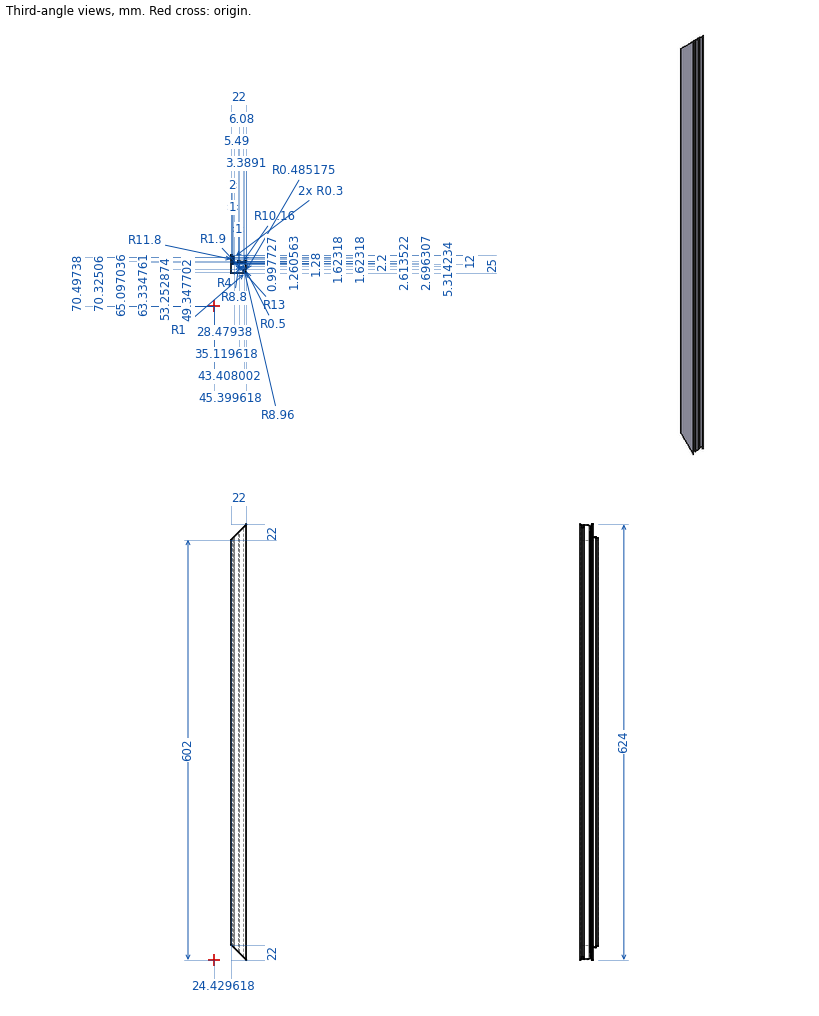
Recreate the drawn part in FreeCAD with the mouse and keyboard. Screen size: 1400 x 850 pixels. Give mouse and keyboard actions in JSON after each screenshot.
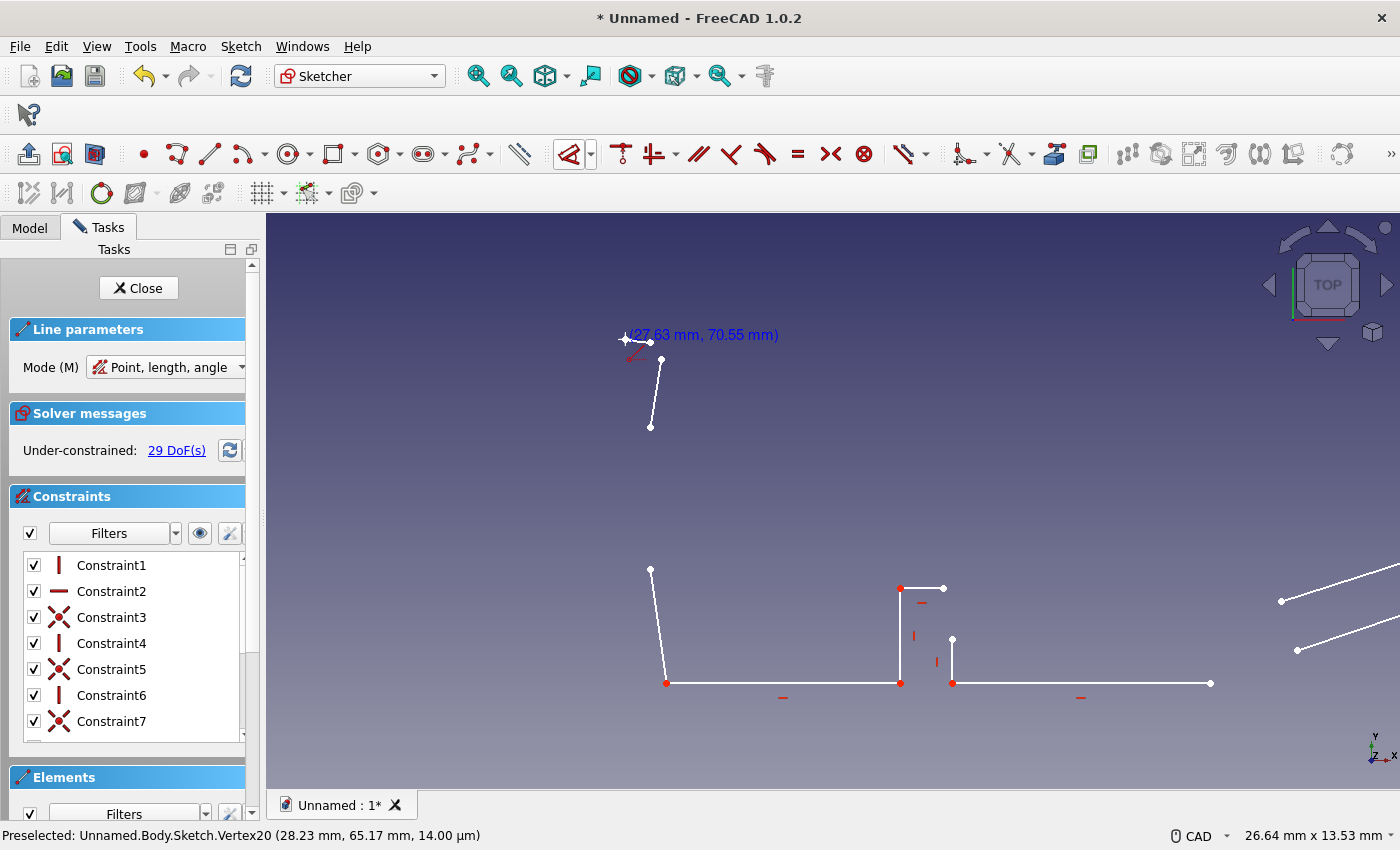
{"action": "left_click", "coordinate": [611, 350]}
{"action": "left_click", "coordinate": [601, 419]}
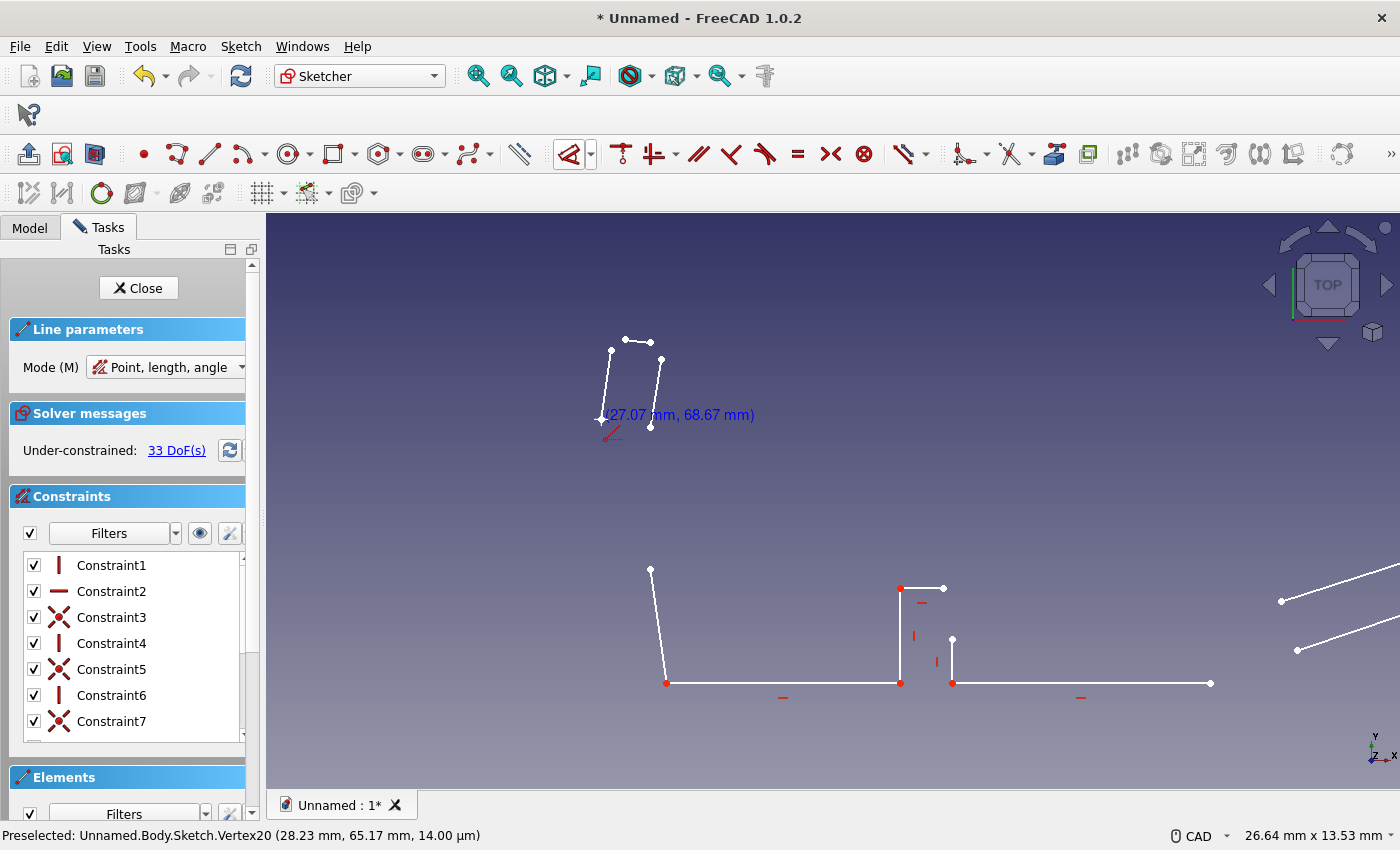
{"action": "key", "text": "g m"}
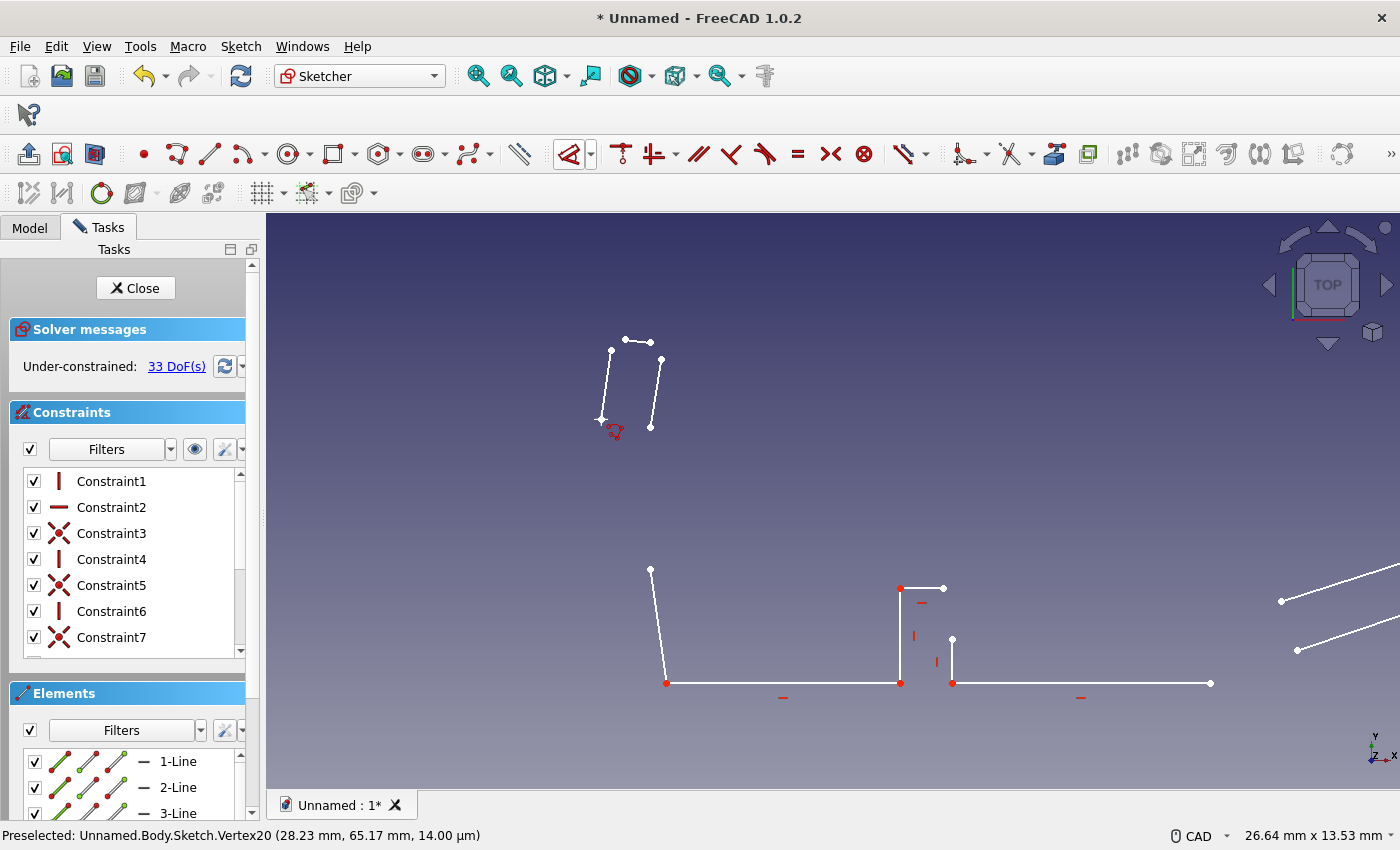
{"action": "left_click", "coordinate": [601, 572]}
{"action": "left_click", "coordinate": [616, 684]}
{"action": "left_click", "coordinate": [616, 738]}
{"action": "left_click", "coordinate": [574, 738]}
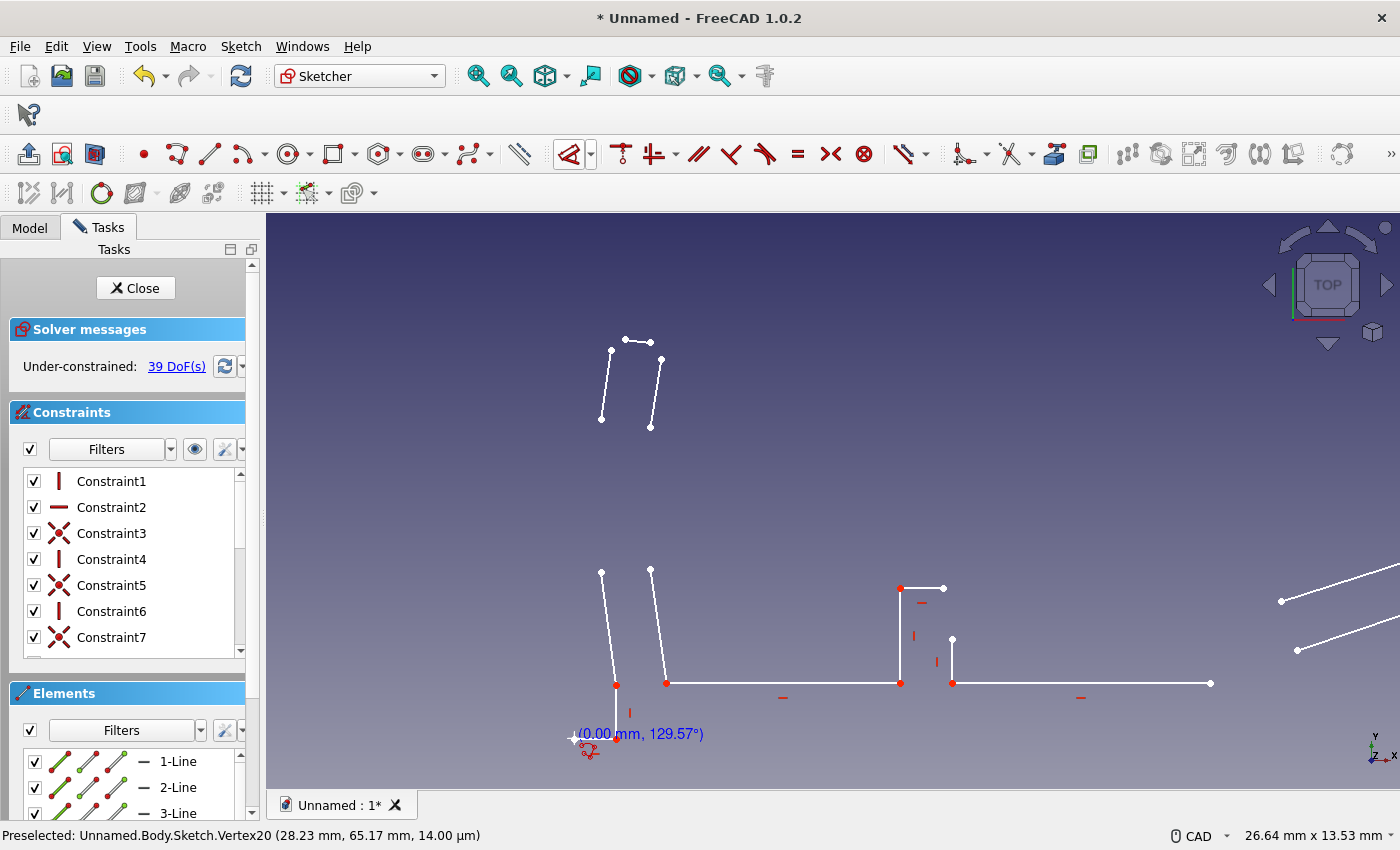
{"action": "scroll", "coordinate": [653, 351], "scroll_direction": "down", "scroll_amount": 5}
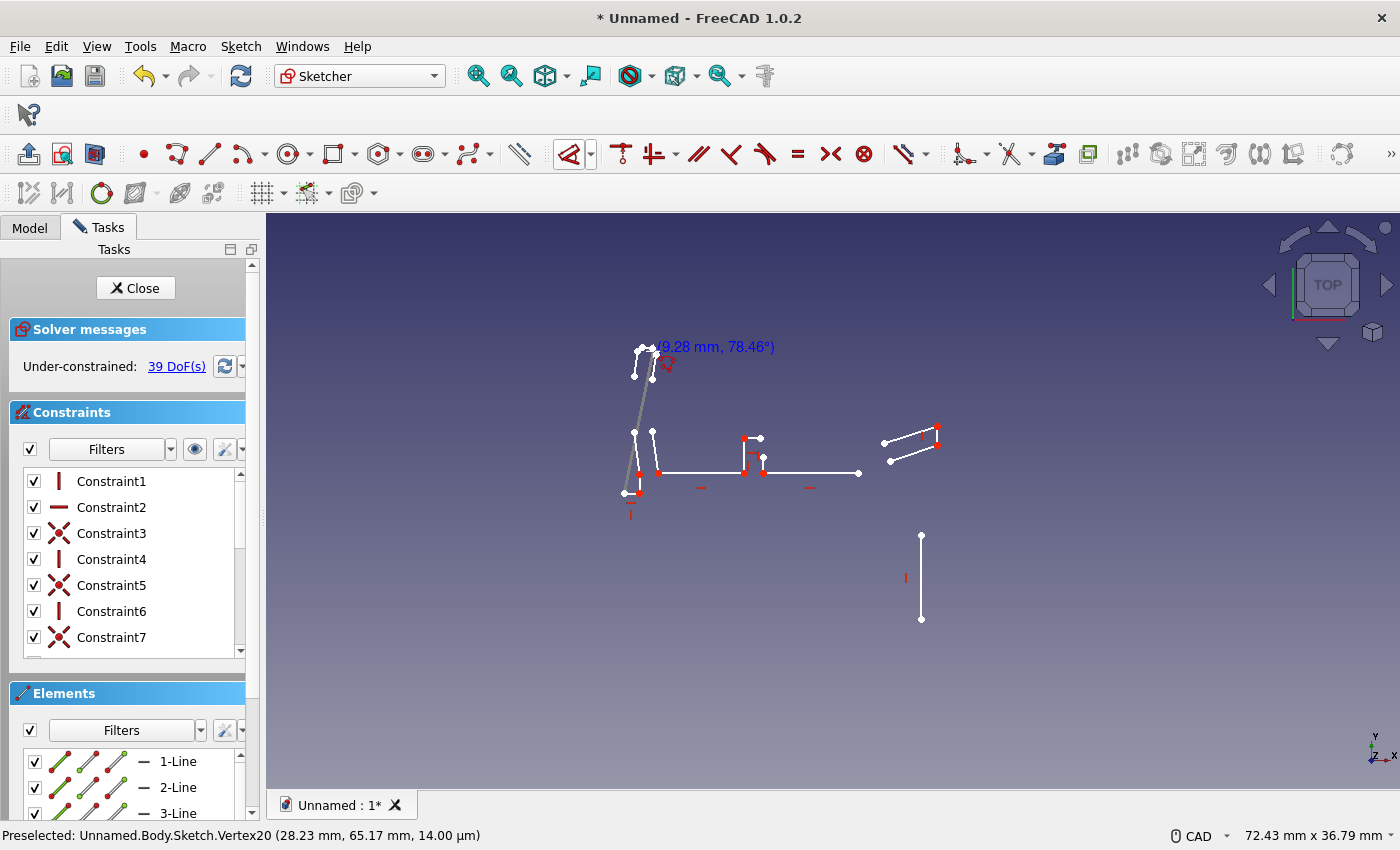
{"action": "left_click", "coordinate": [624, 306]}
{"action": "left_click", "coordinate": [593, 306]}
{"action": "left_click", "coordinate": [593, 697]}
{"action": "left_click", "coordinate": [937, 697]}
{"action": "right_click", "coordinate": [937, 697]}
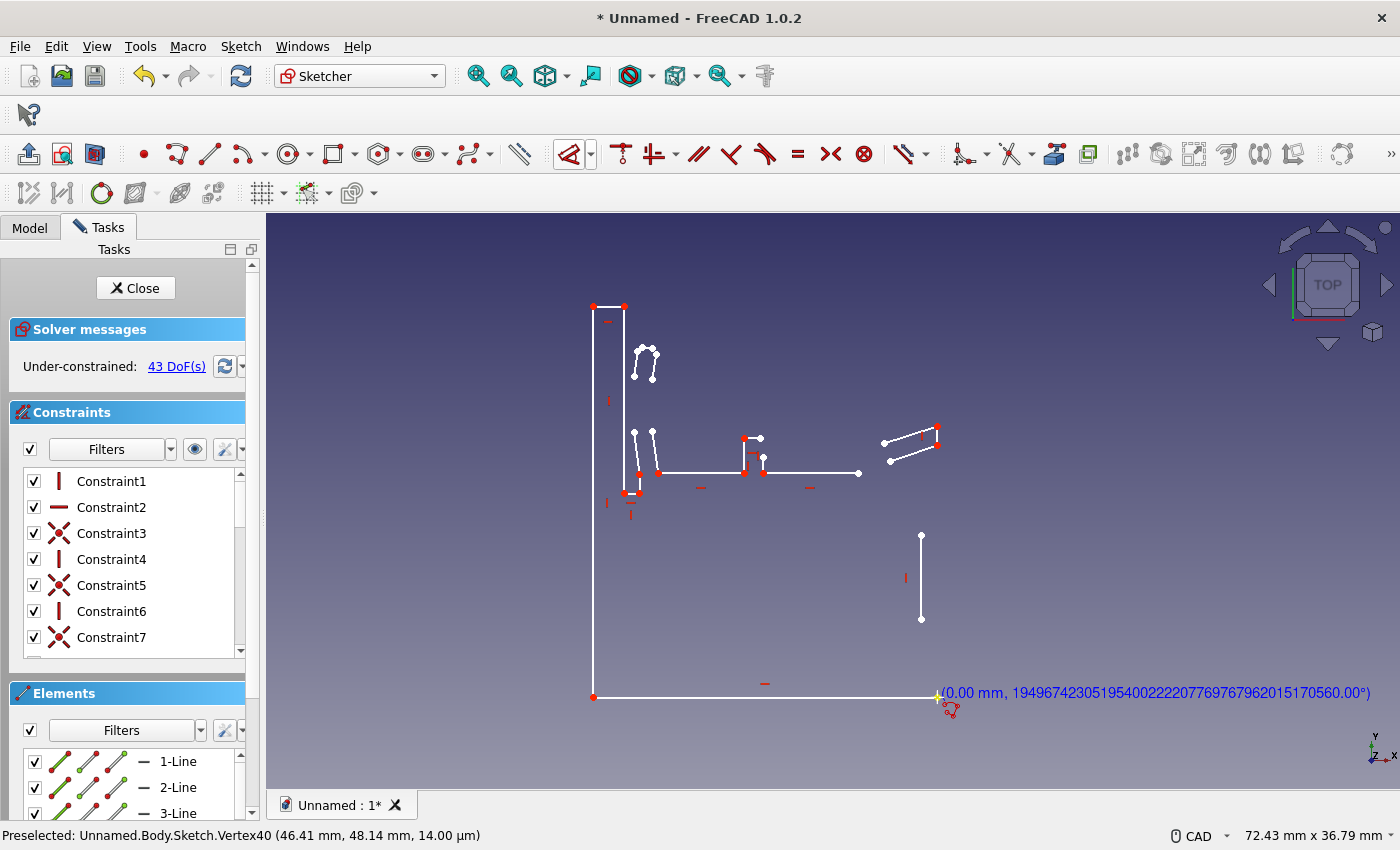
{"action": "key", "text": "g 3 a"}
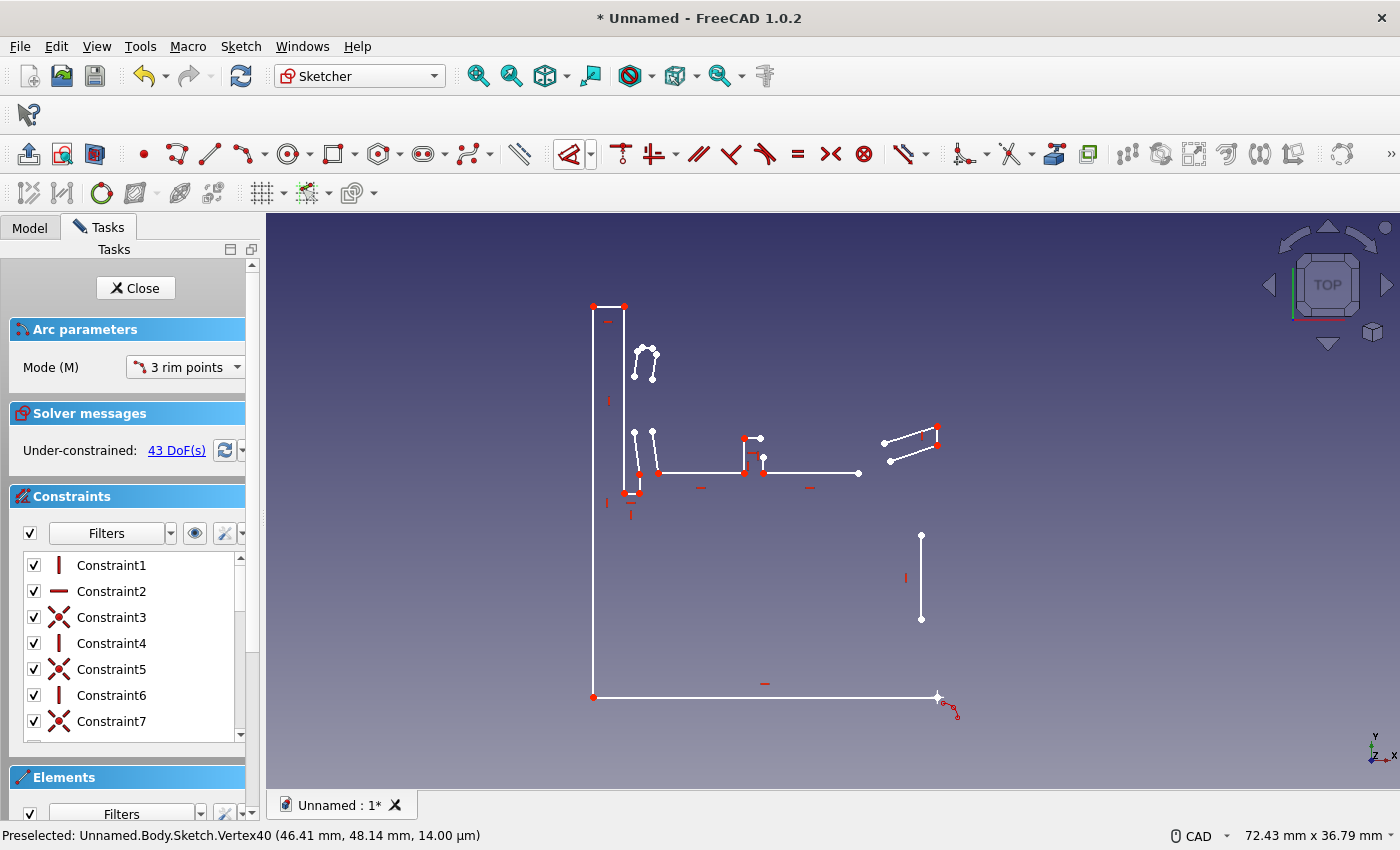
{"action": "left_click", "coordinate": [921, 535]}
{"action": "left_click", "coordinate": [858, 473]}
{"action": "left_click", "coordinate": [903, 491]}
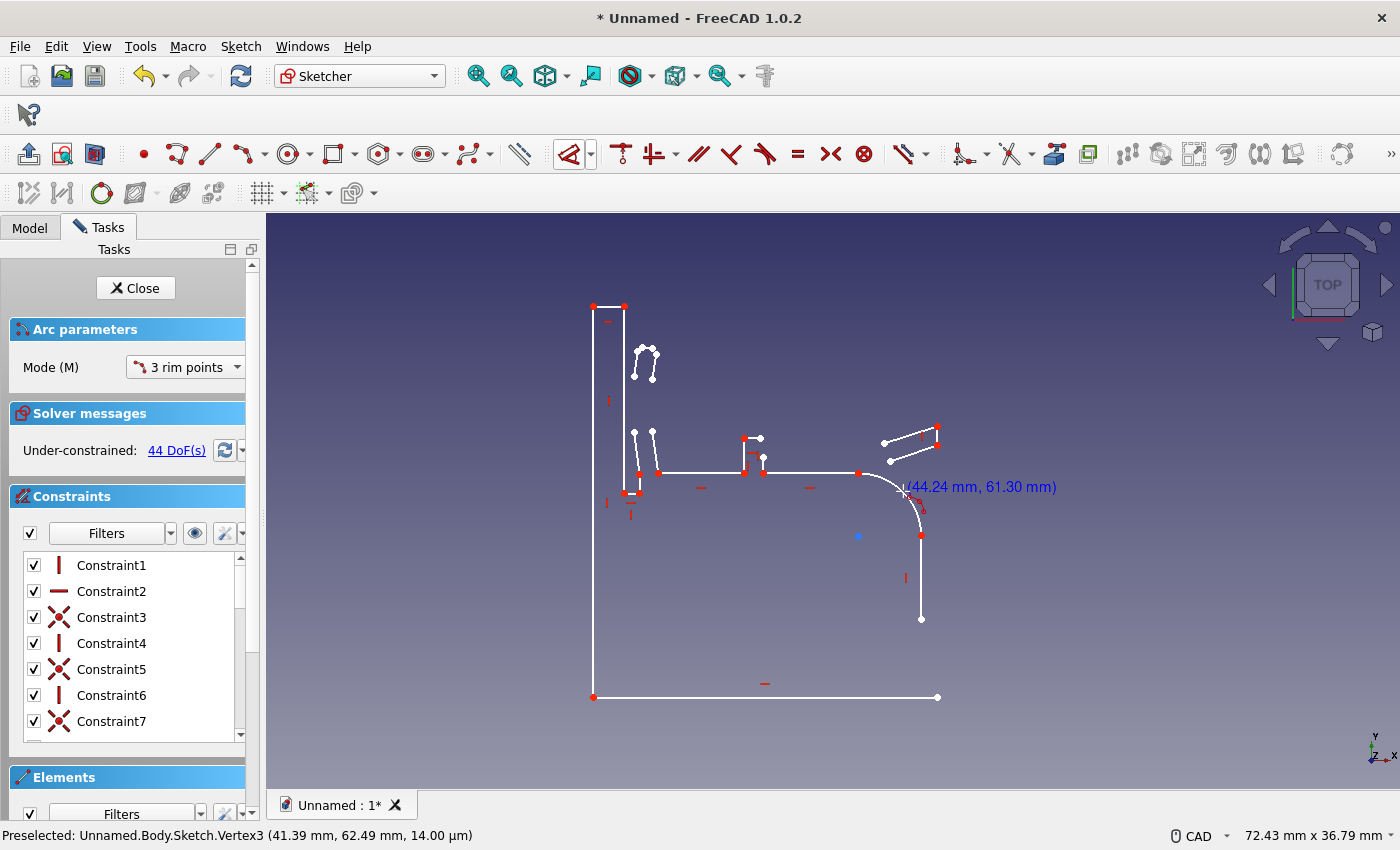
{"action": "scroll", "coordinate": [763, 457], "scroll_direction": "up", "scroll_amount": 4}